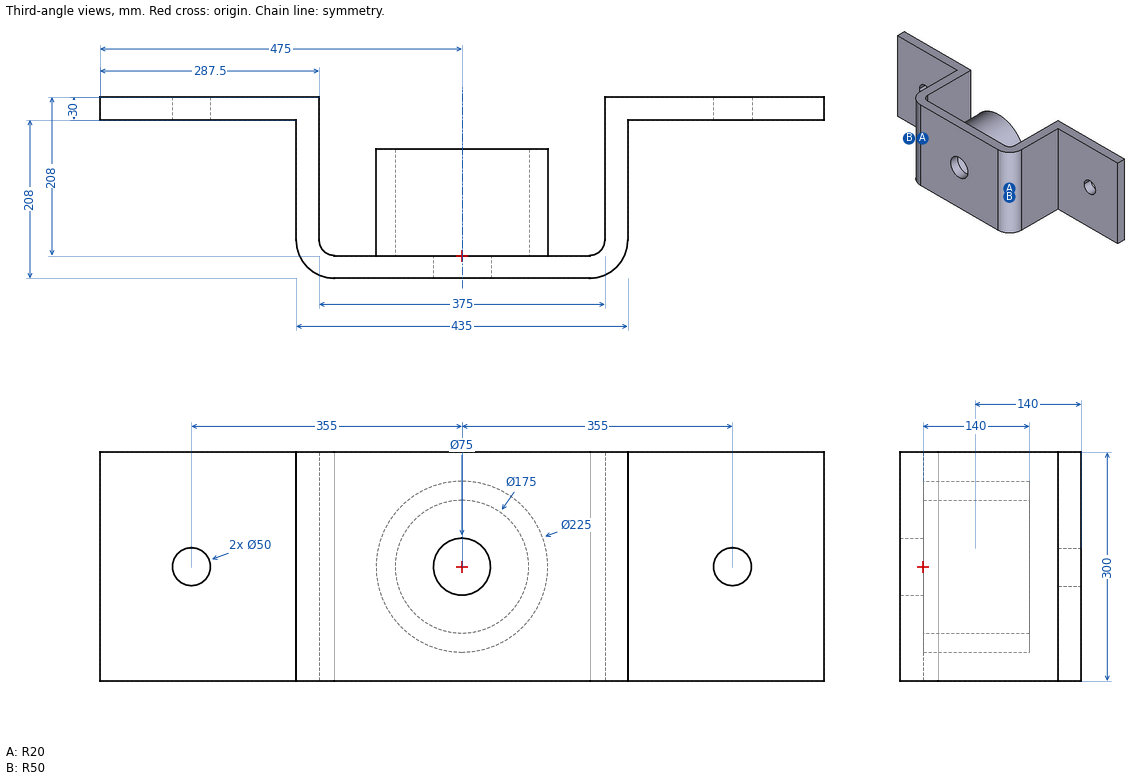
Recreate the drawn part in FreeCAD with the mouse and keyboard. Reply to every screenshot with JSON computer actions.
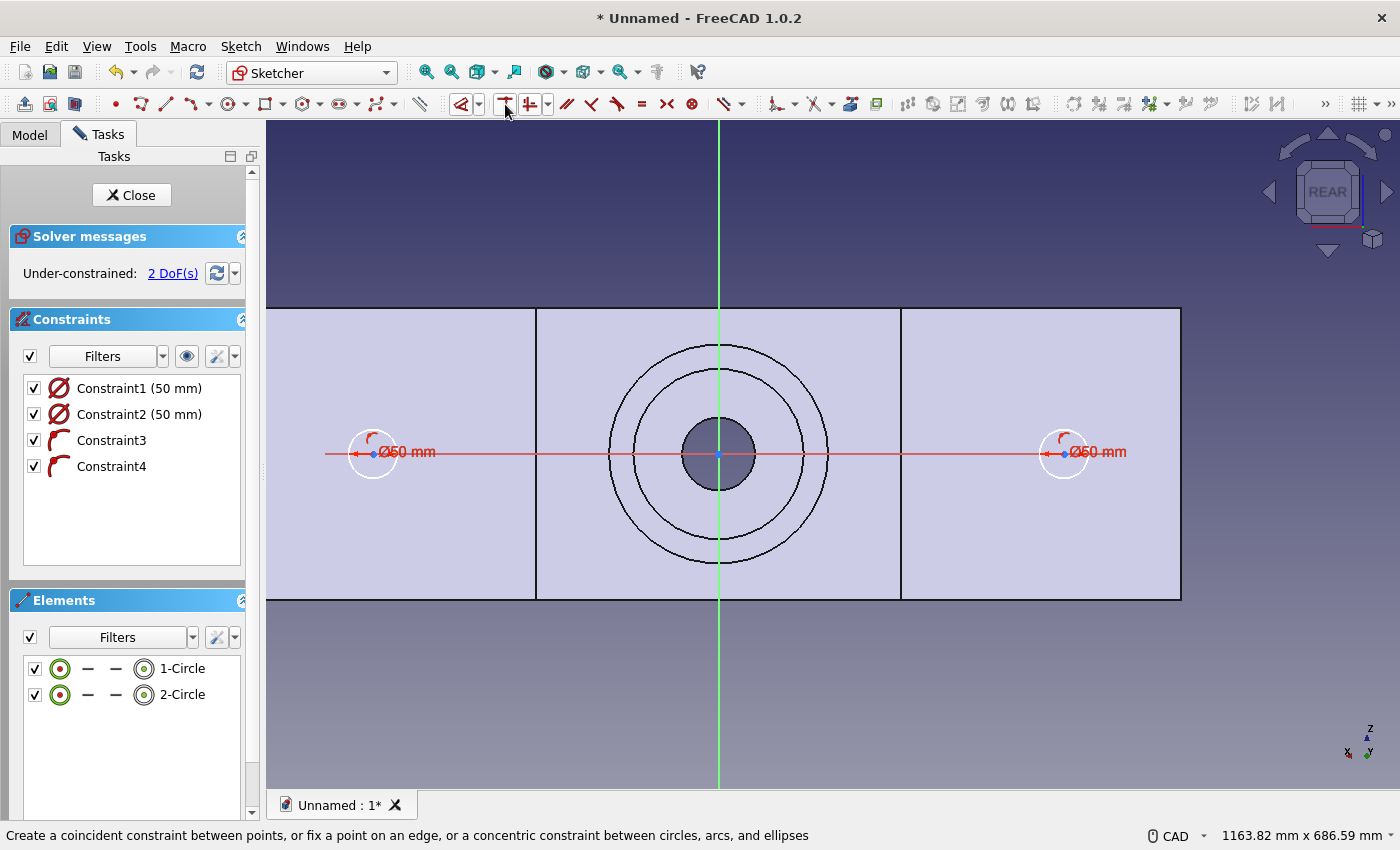
{"action": "left_click", "coordinate": [1064, 454]}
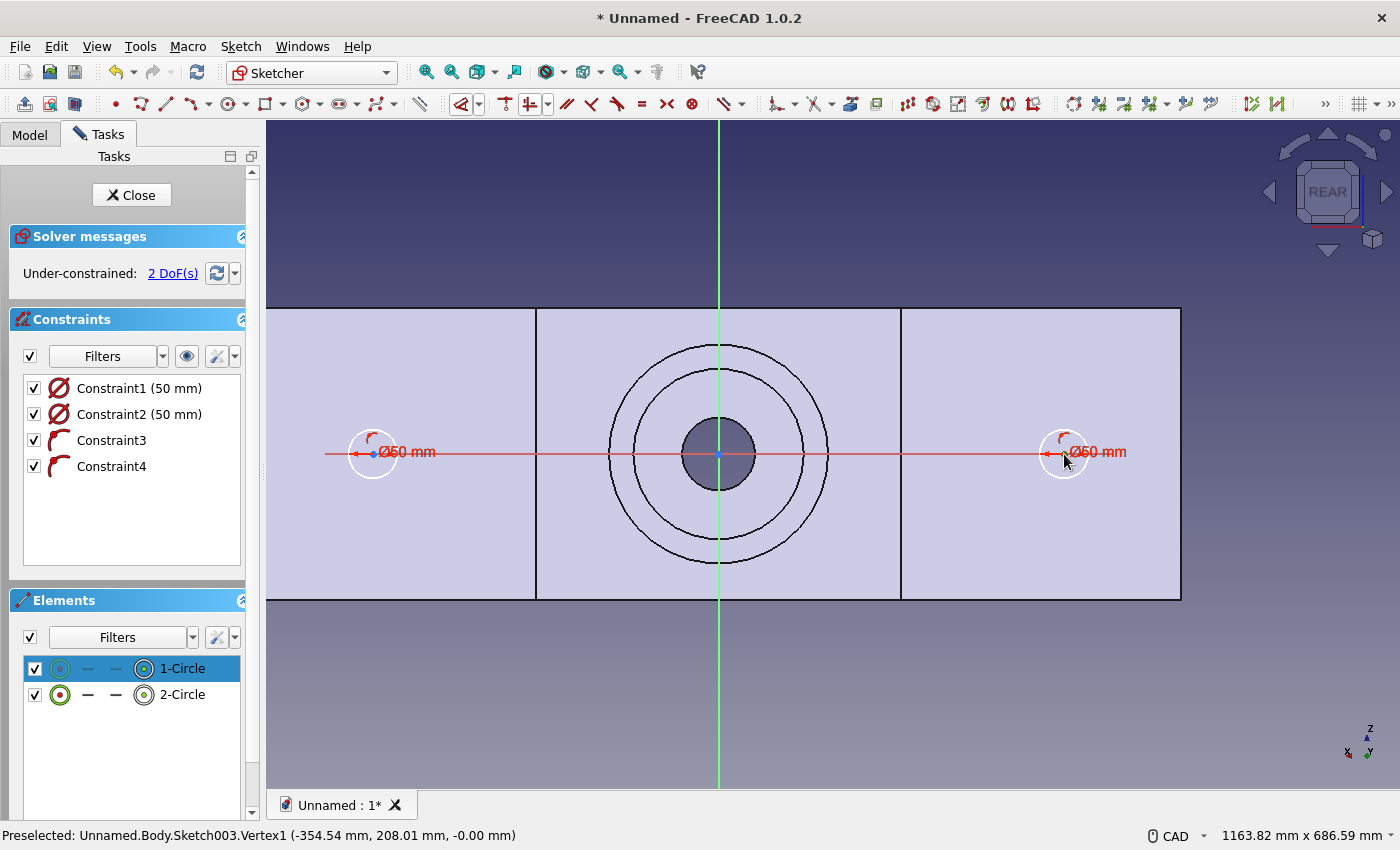
{"action": "key", "text": "l"}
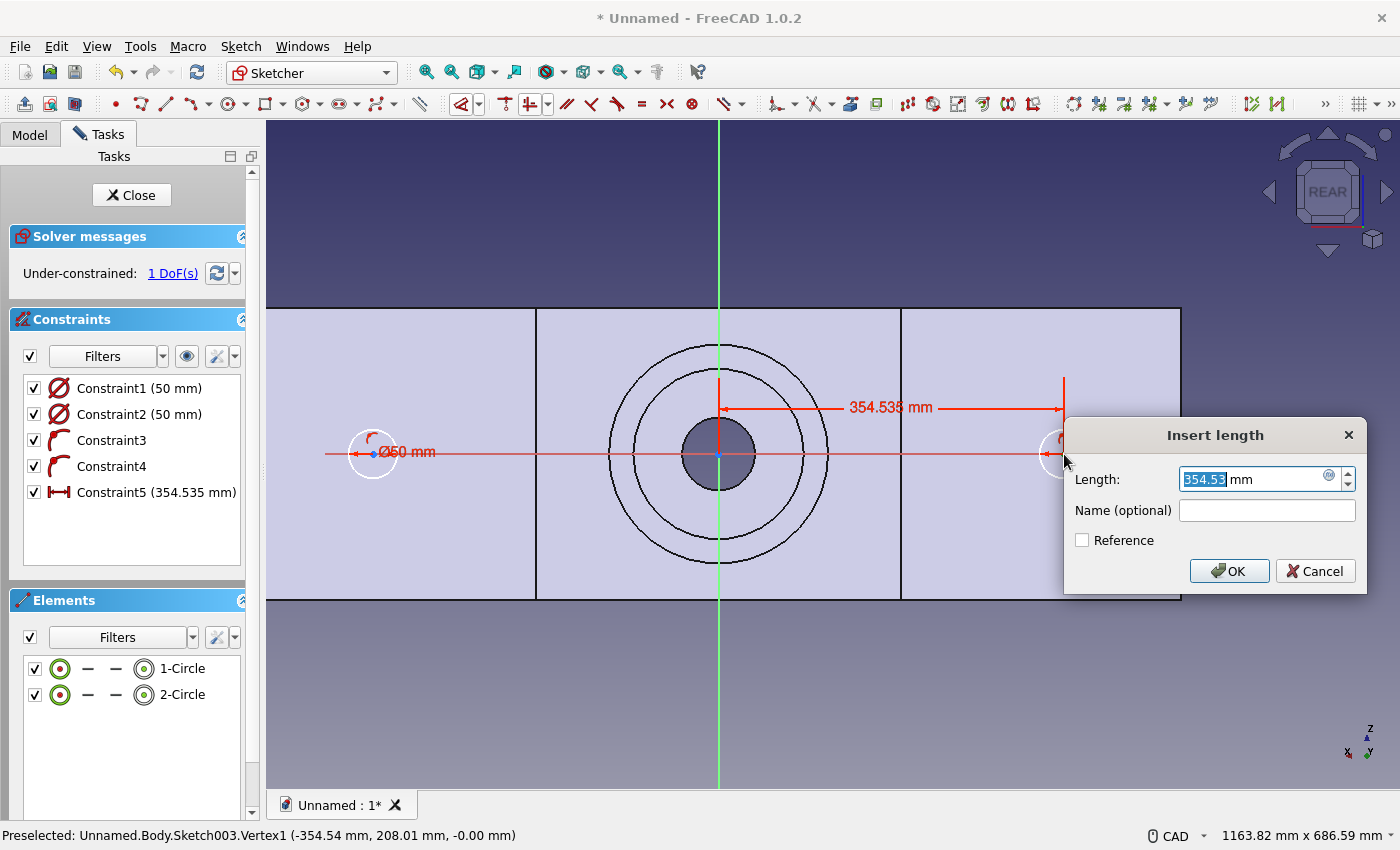
{"action": "type", "text": "355"}
{"action": "key", "text": "Return"}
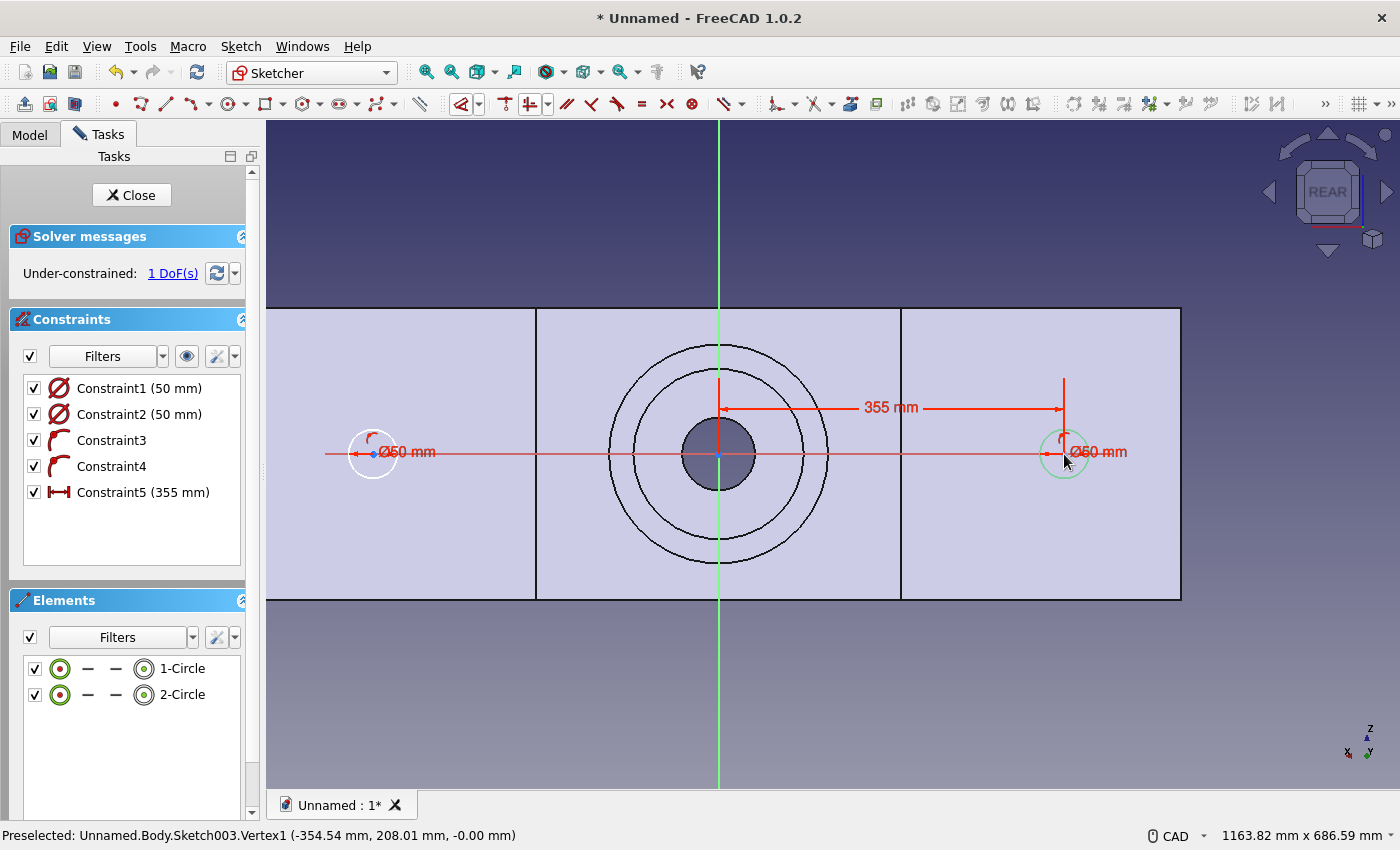
{"action": "left_click", "coordinate": [373, 454]}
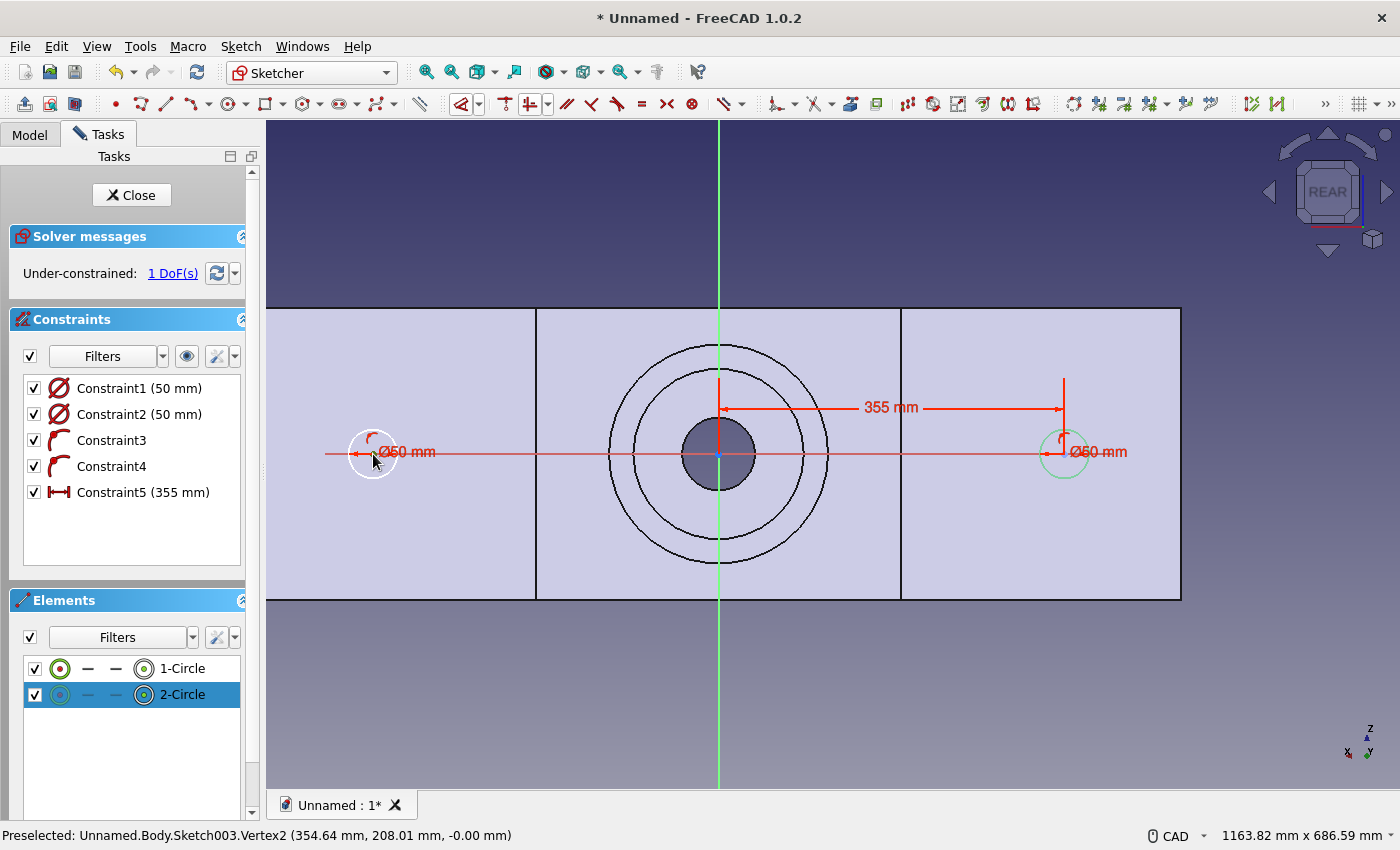
{"action": "left_click", "coordinate": [478, 104]}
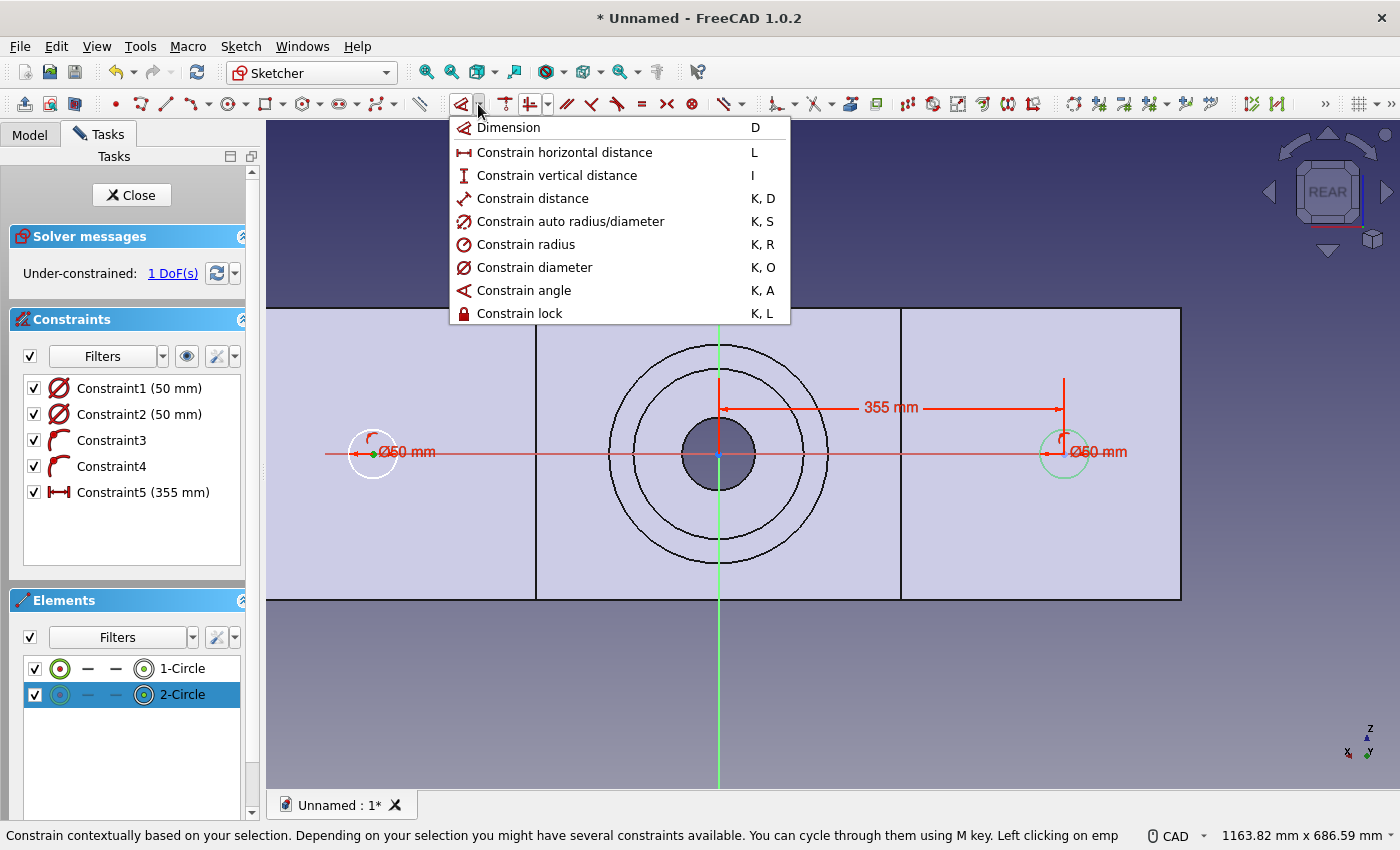
{"action": "left_click", "coordinate": [620, 152]}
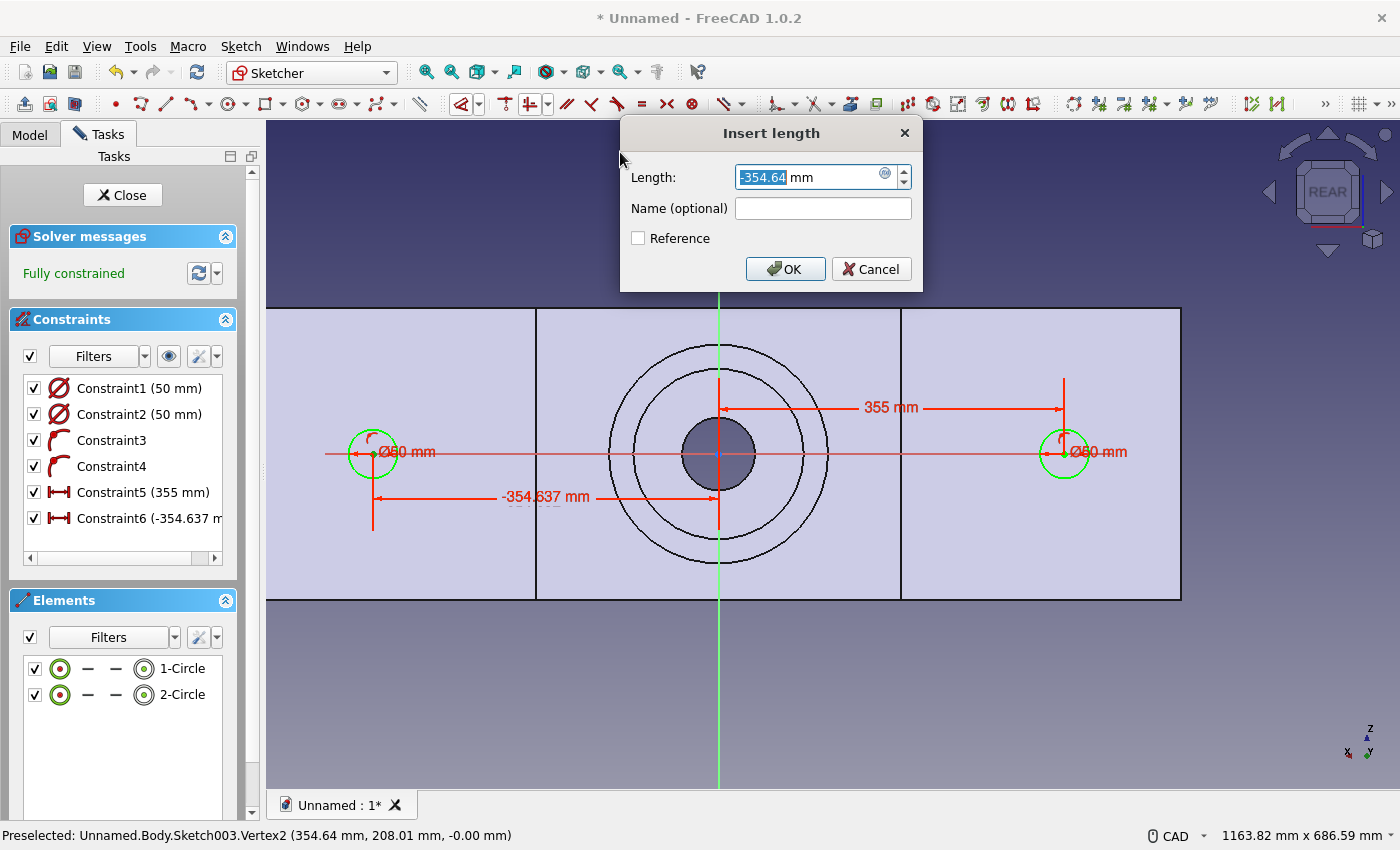
{"action": "type", "text": "-355"}
{"action": "key", "text": "Return"}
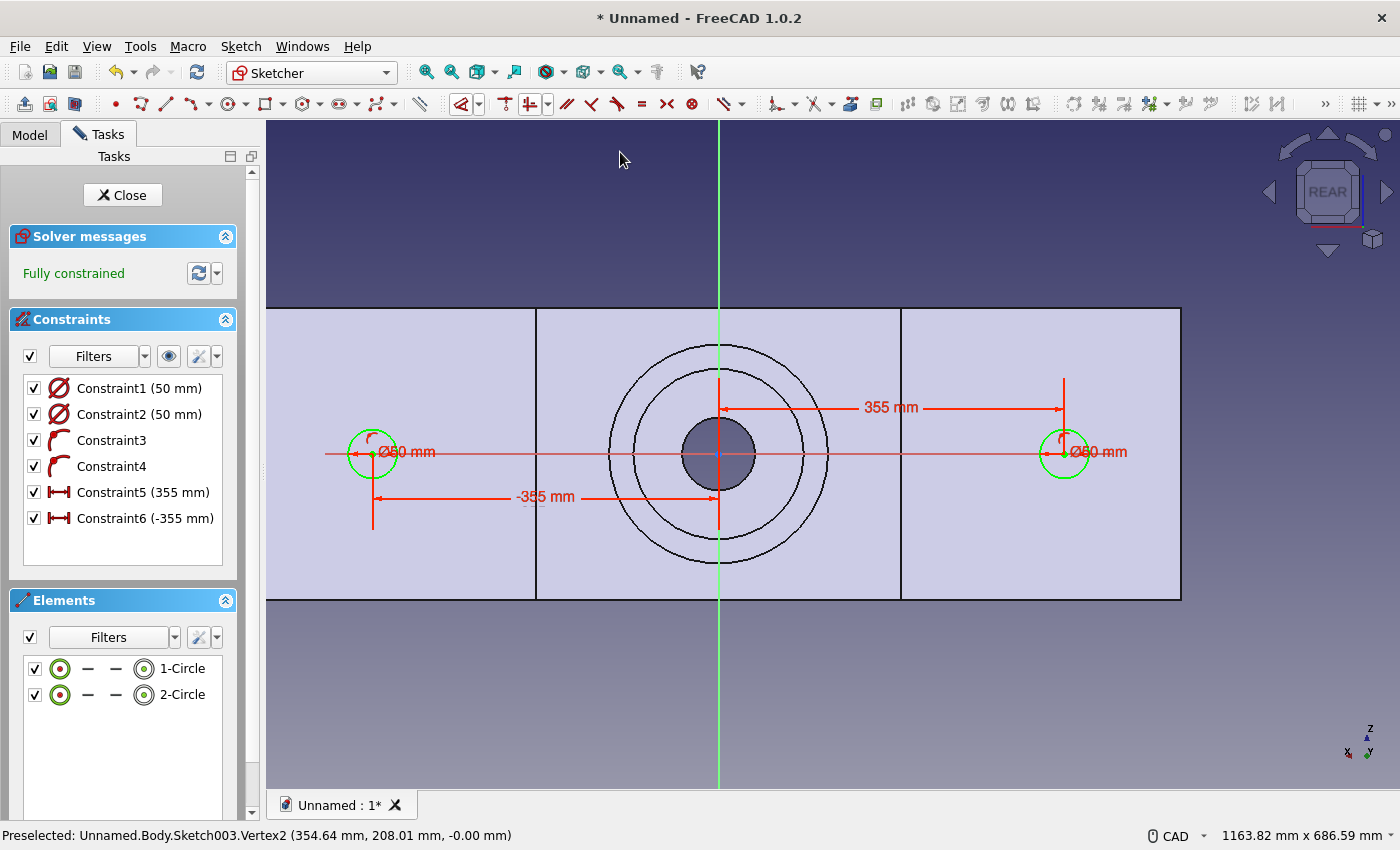
{"action": "left_click", "coordinate": [123, 195]}